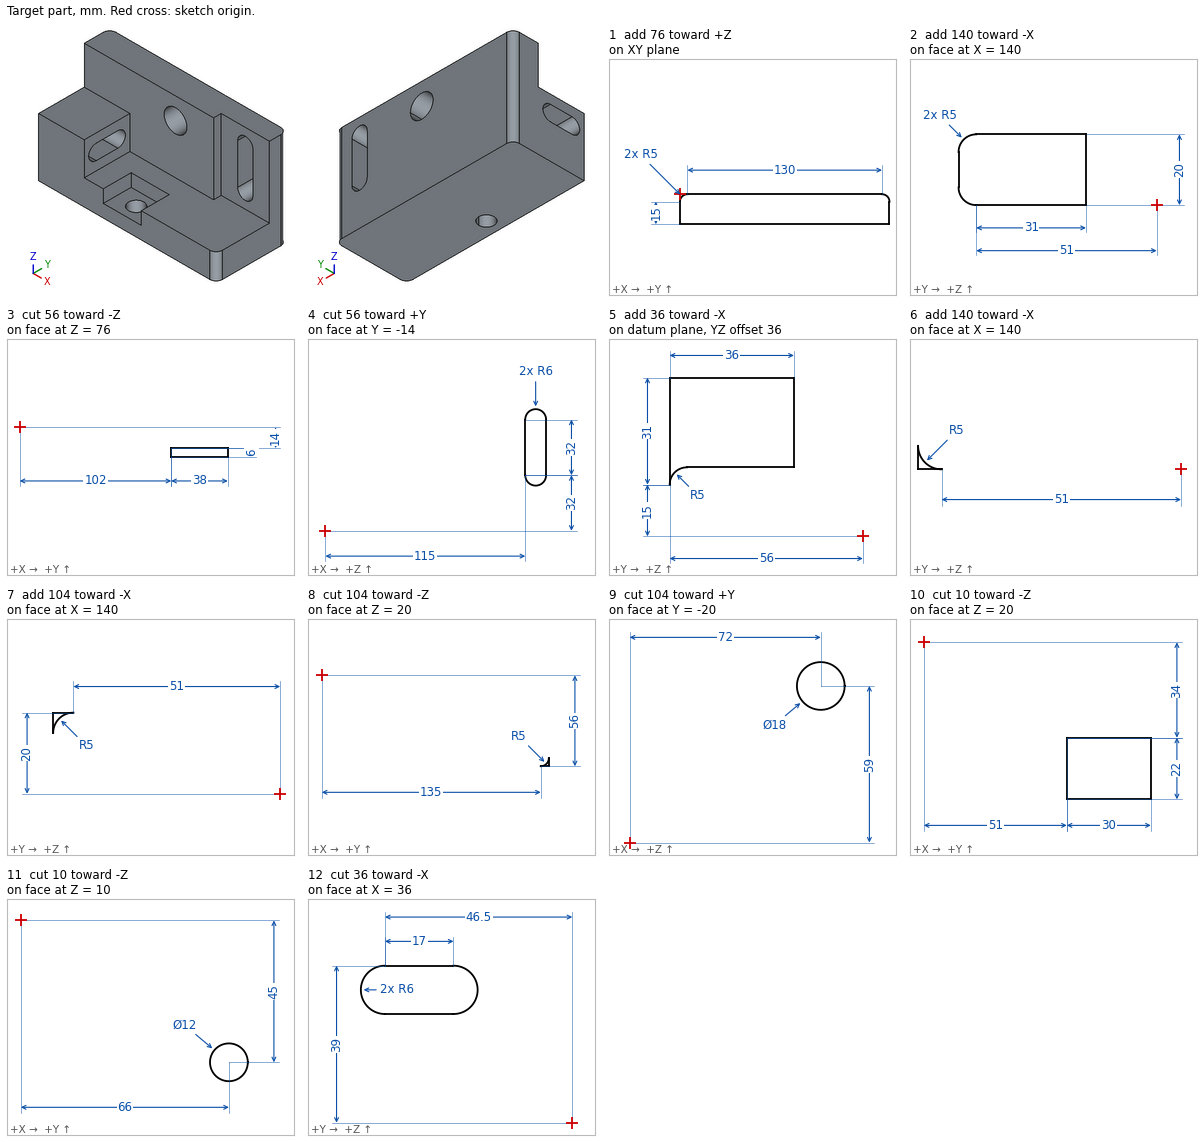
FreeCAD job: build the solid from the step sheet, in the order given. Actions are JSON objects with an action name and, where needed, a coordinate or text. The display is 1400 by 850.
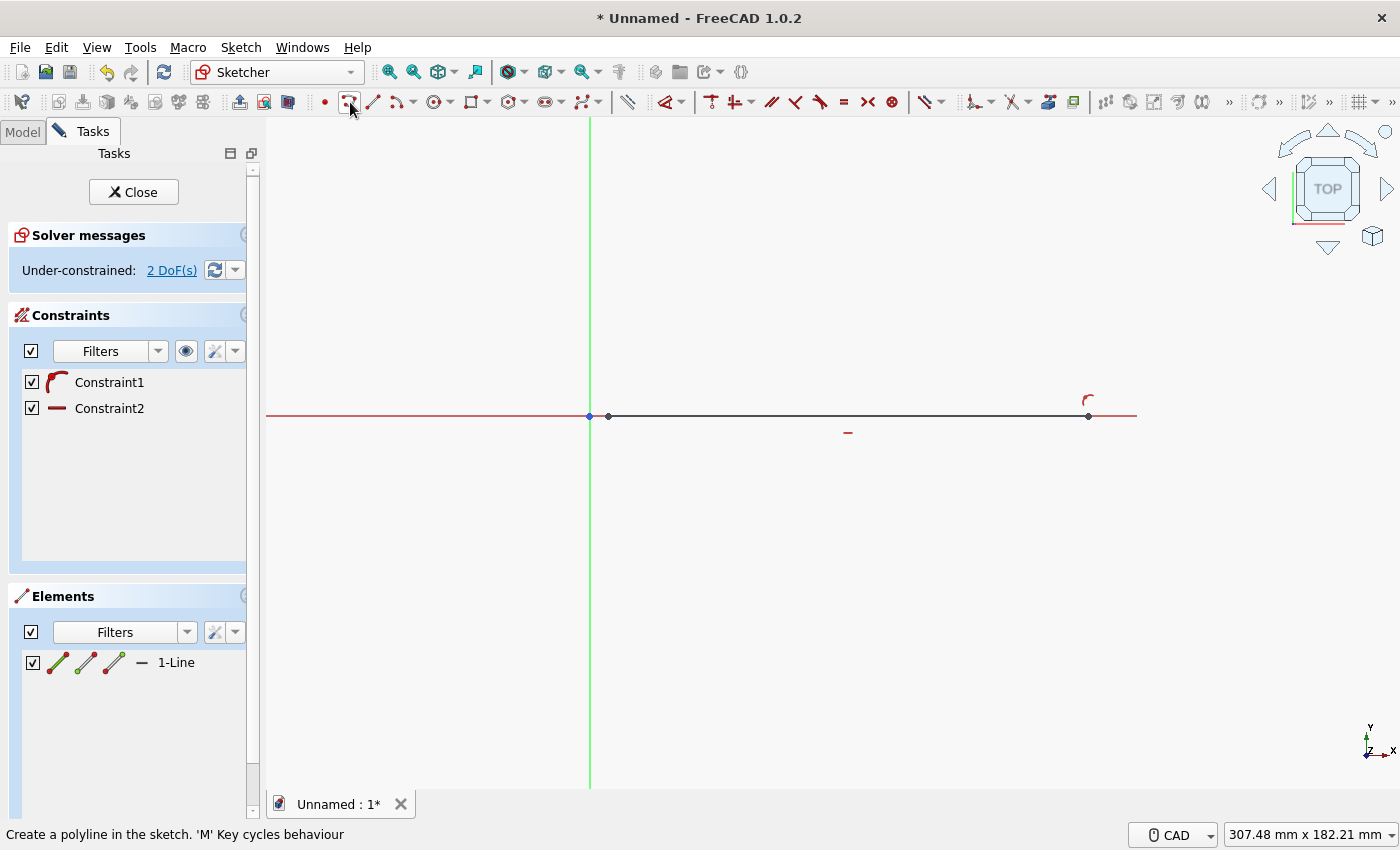
{"action": "left_click", "coordinate": [590, 435]}
{"action": "left_click", "coordinate": [599, 490]}
{"action": "left_click", "coordinate": [1106, 490]}
{"action": "left_click", "coordinate": [1106, 435]}
{"action": "right_click", "coordinate": [1106, 435]}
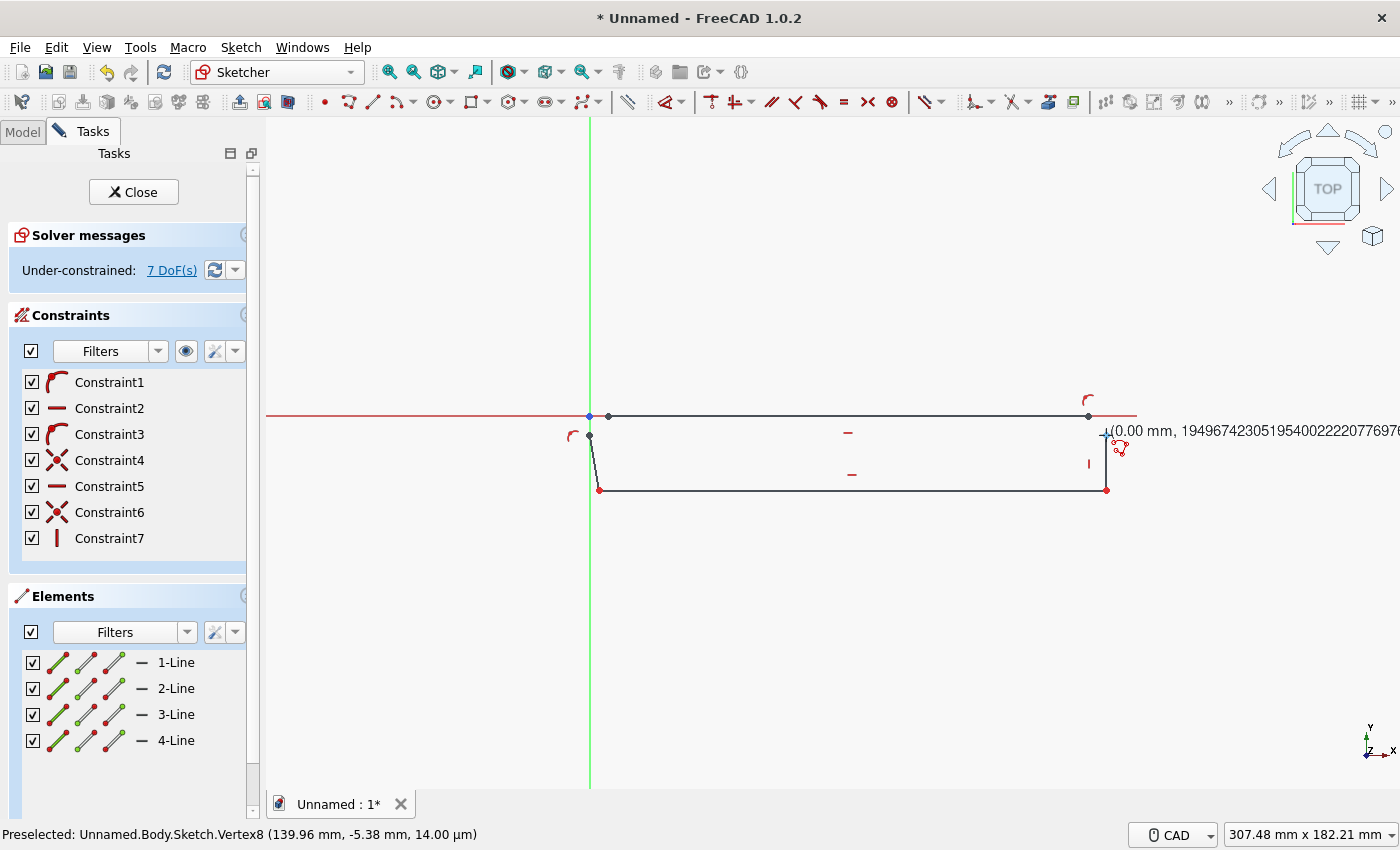
{"action": "key", "text": "g 3 a"}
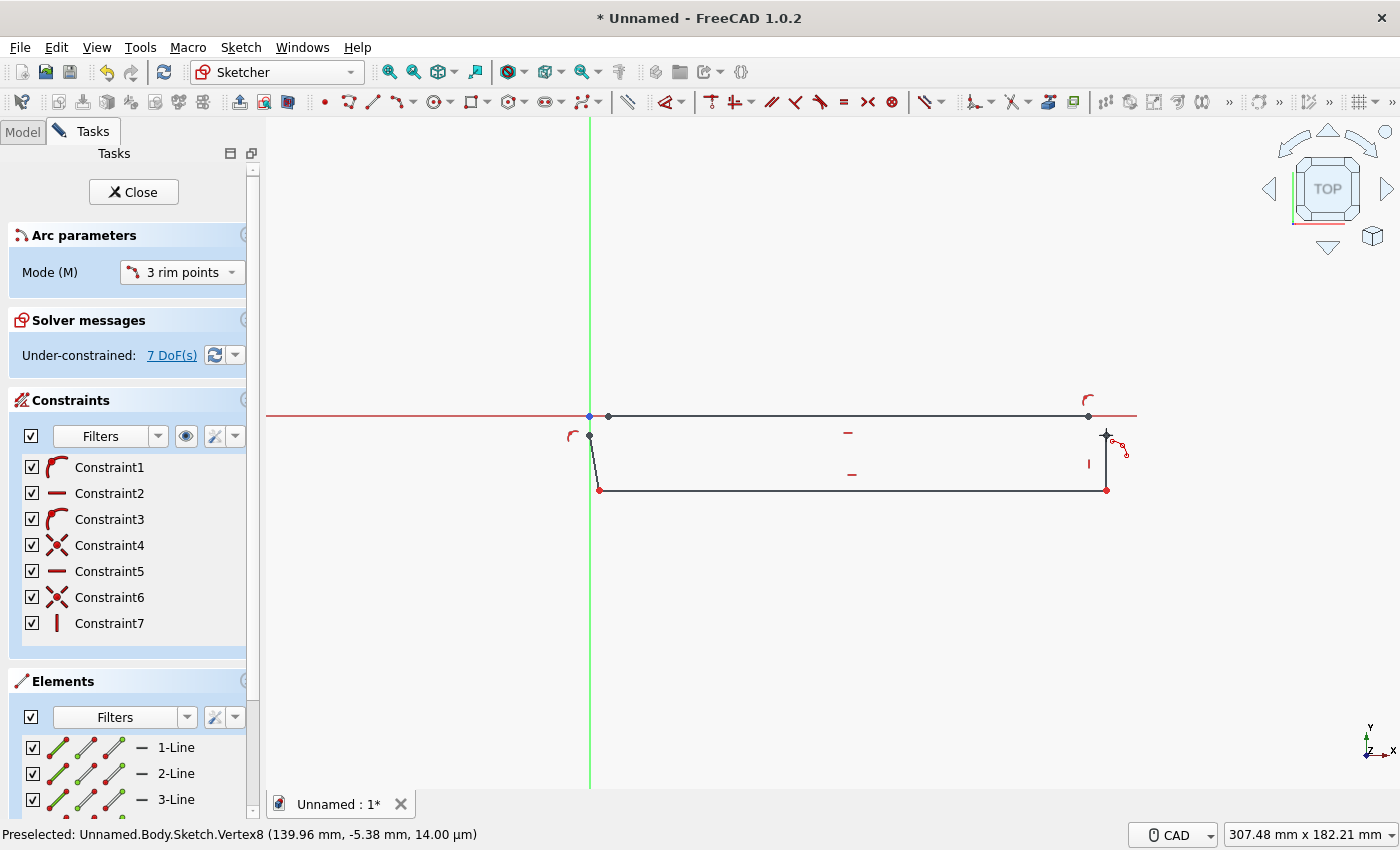
{"action": "left_click", "coordinate": [608, 416]}
{"action": "left_click", "coordinate": [590, 436]}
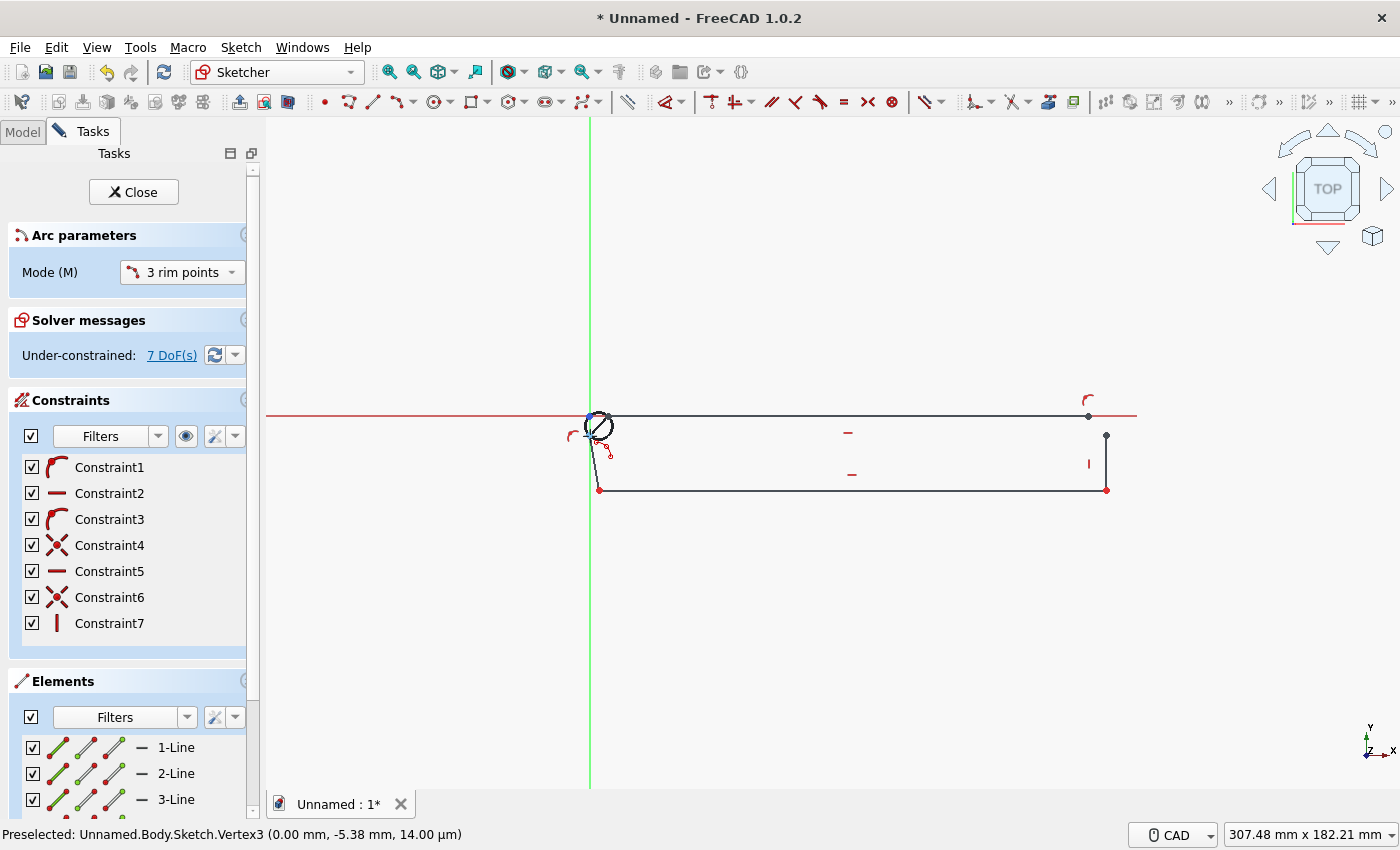
{"action": "scroll", "coordinate": [595, 422], "scroll_direction": "up", "scroll_amount": 6}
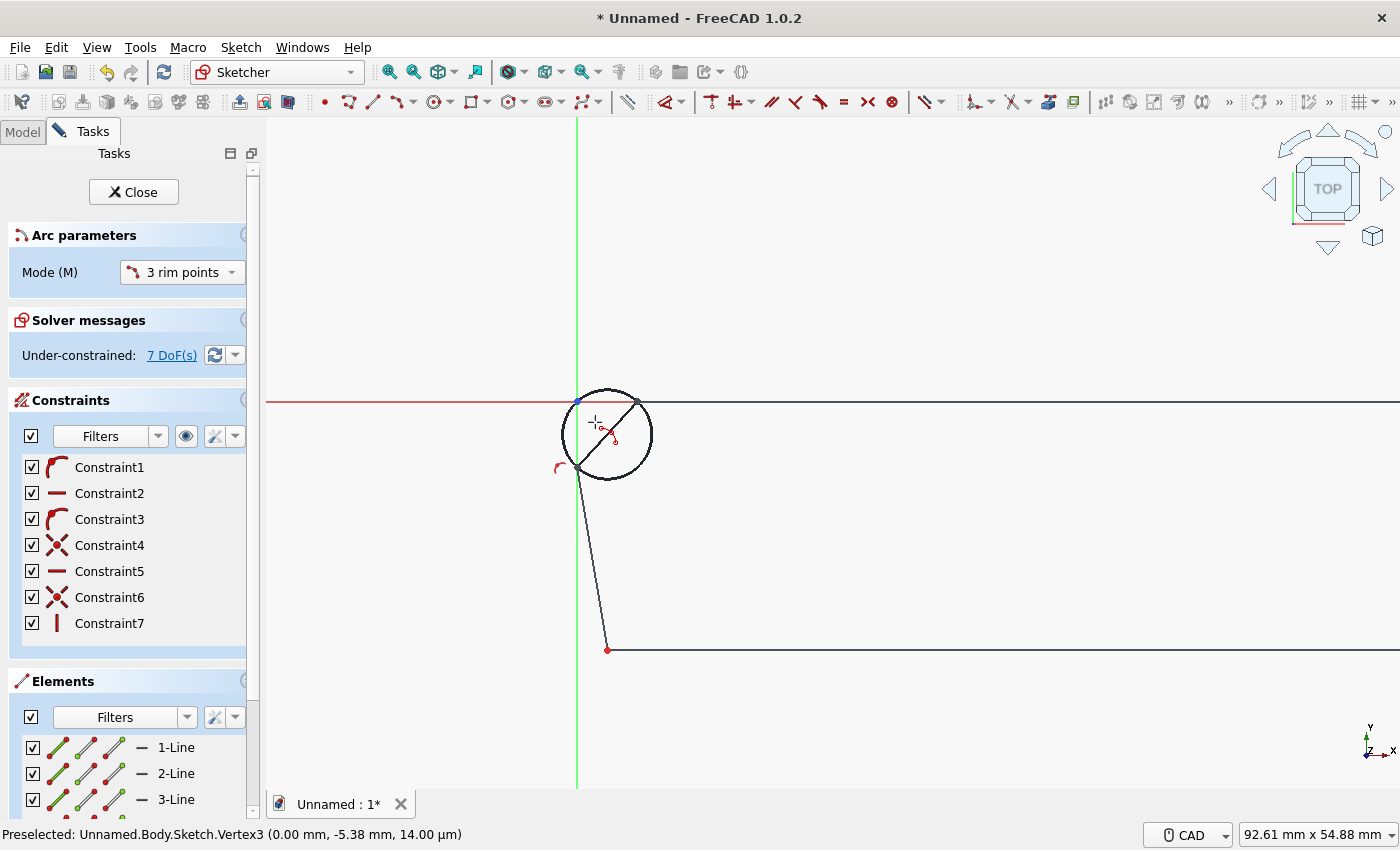
{"action": "left_click", "coordinate": [595, 420]}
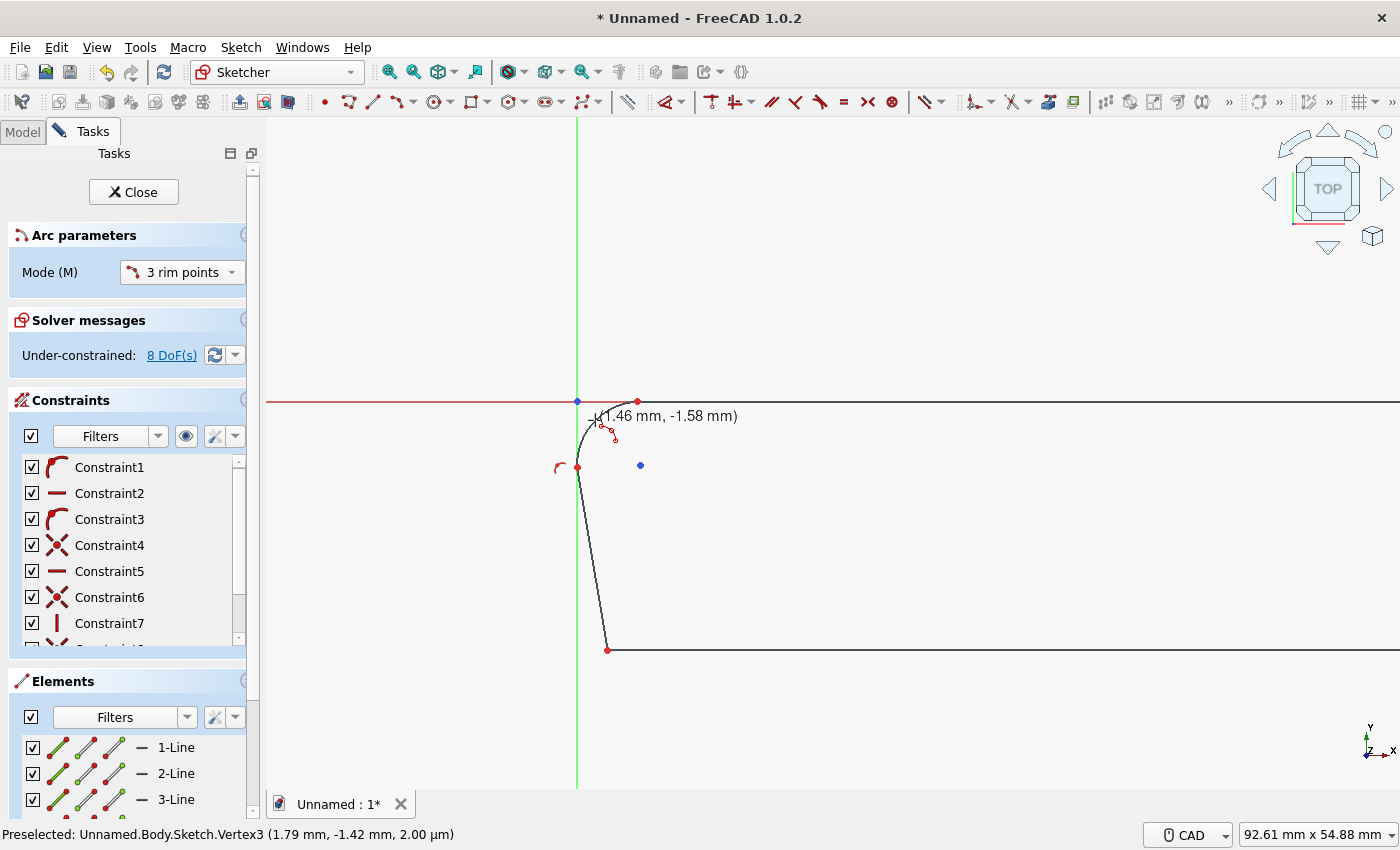
{"action": "scroll", "coordinate": [375, 412], "scroll_direction": "down", "scroll_amount": 5}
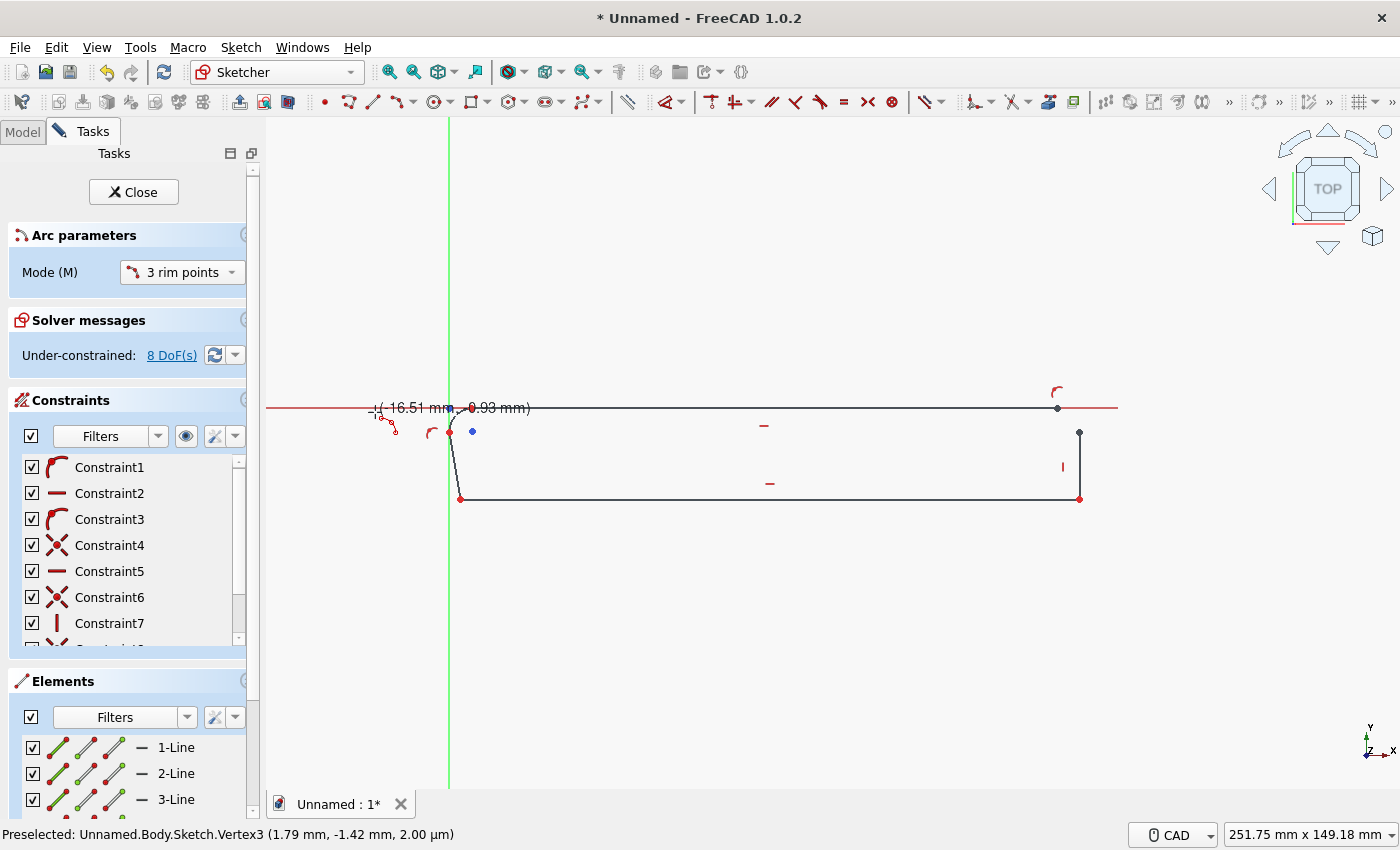
{"action": "left_click", "coordinate": [1080, 433]}
{"action": "left_click", "coordinate": [1058, 408]}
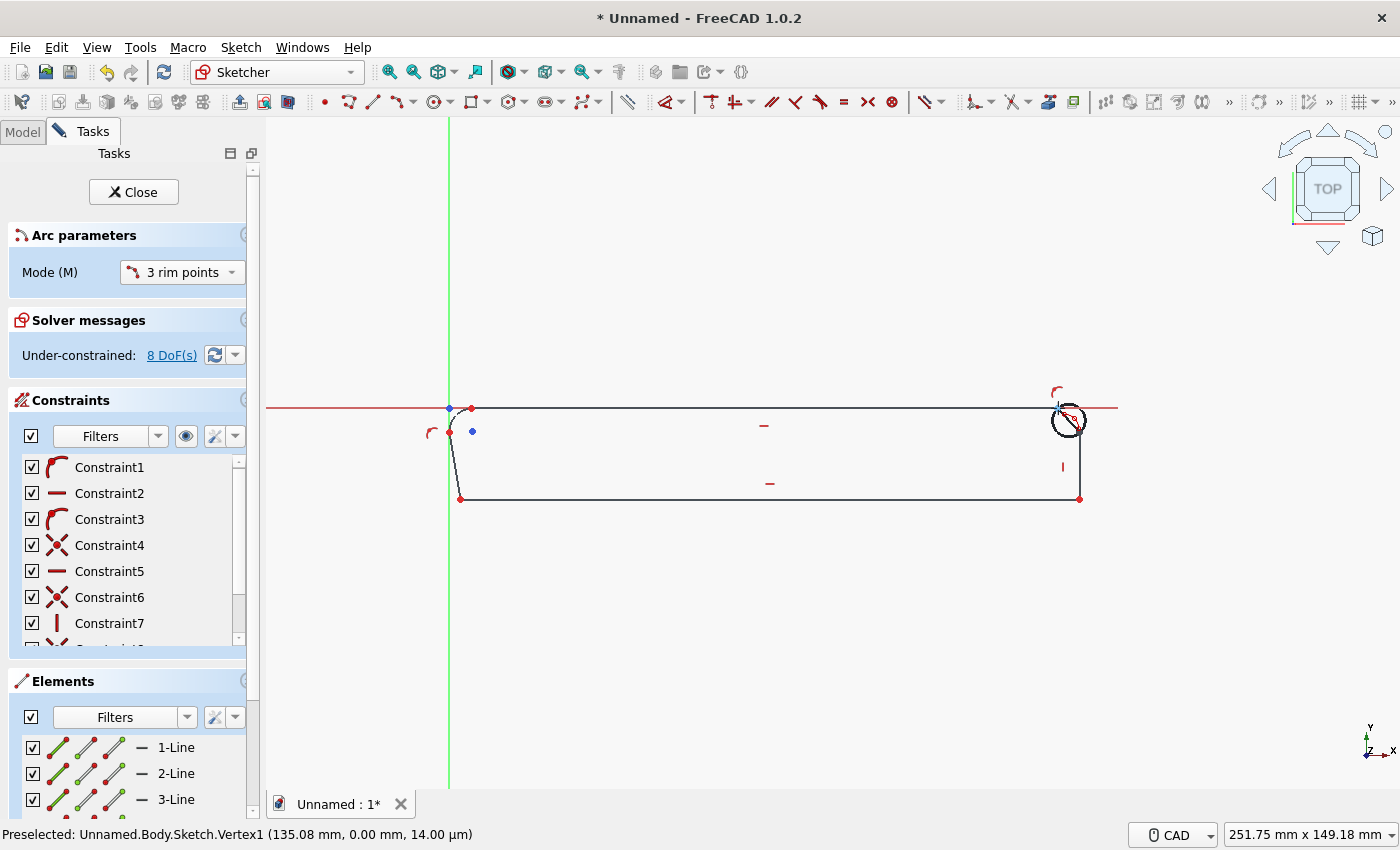
{"action": "scroll", "coordinate": [1073, 415], "scroll_direction": "up", "scroll_amount": 5}